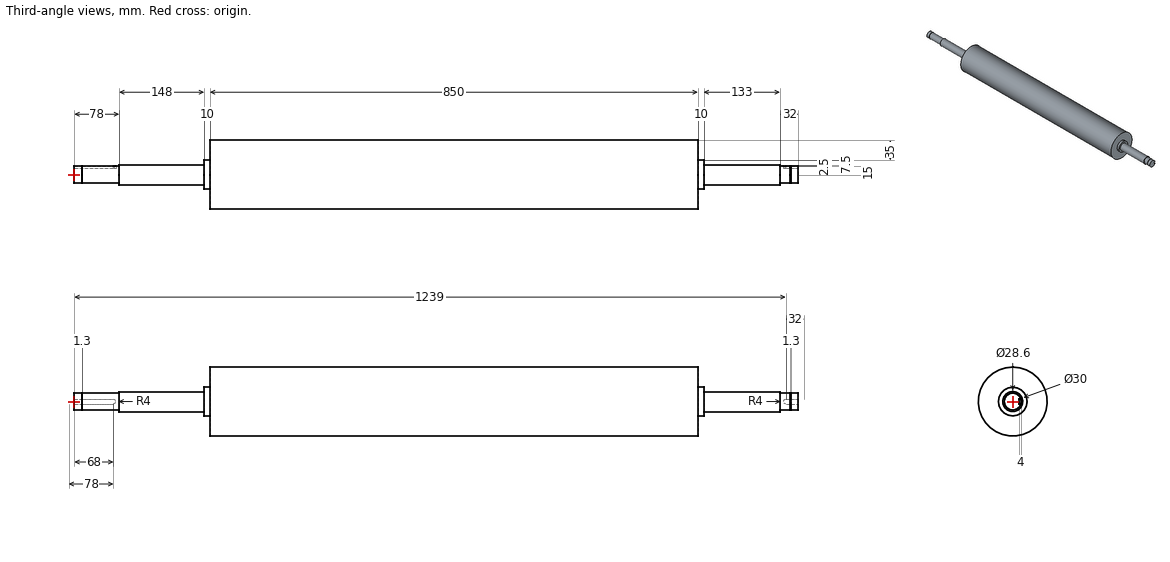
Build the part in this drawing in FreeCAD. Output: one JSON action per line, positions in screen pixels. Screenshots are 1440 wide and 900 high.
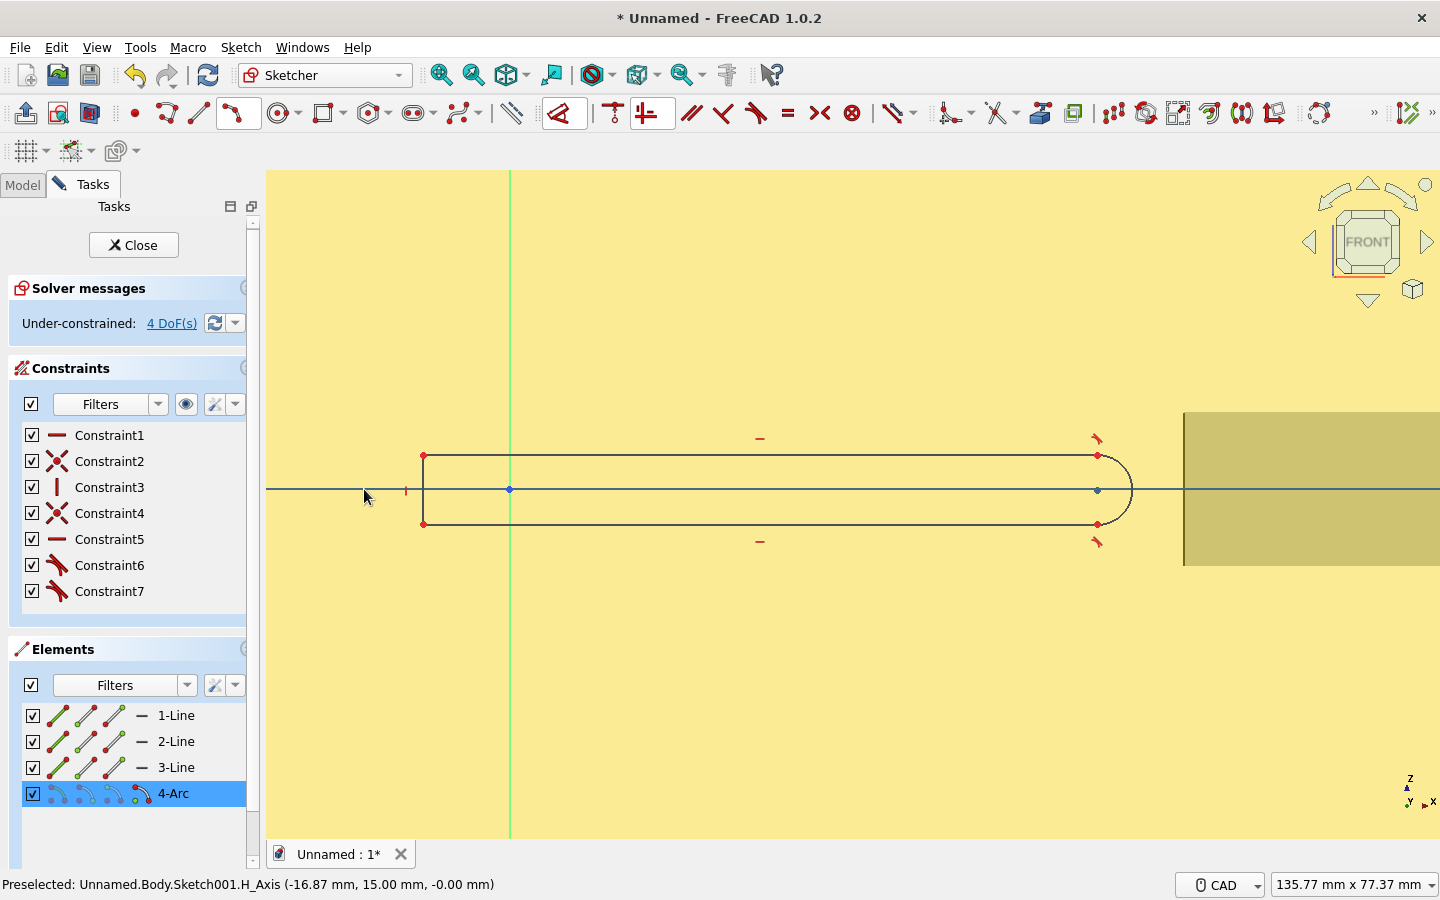
{"action": "left_click", "coordinate": [614, 114]}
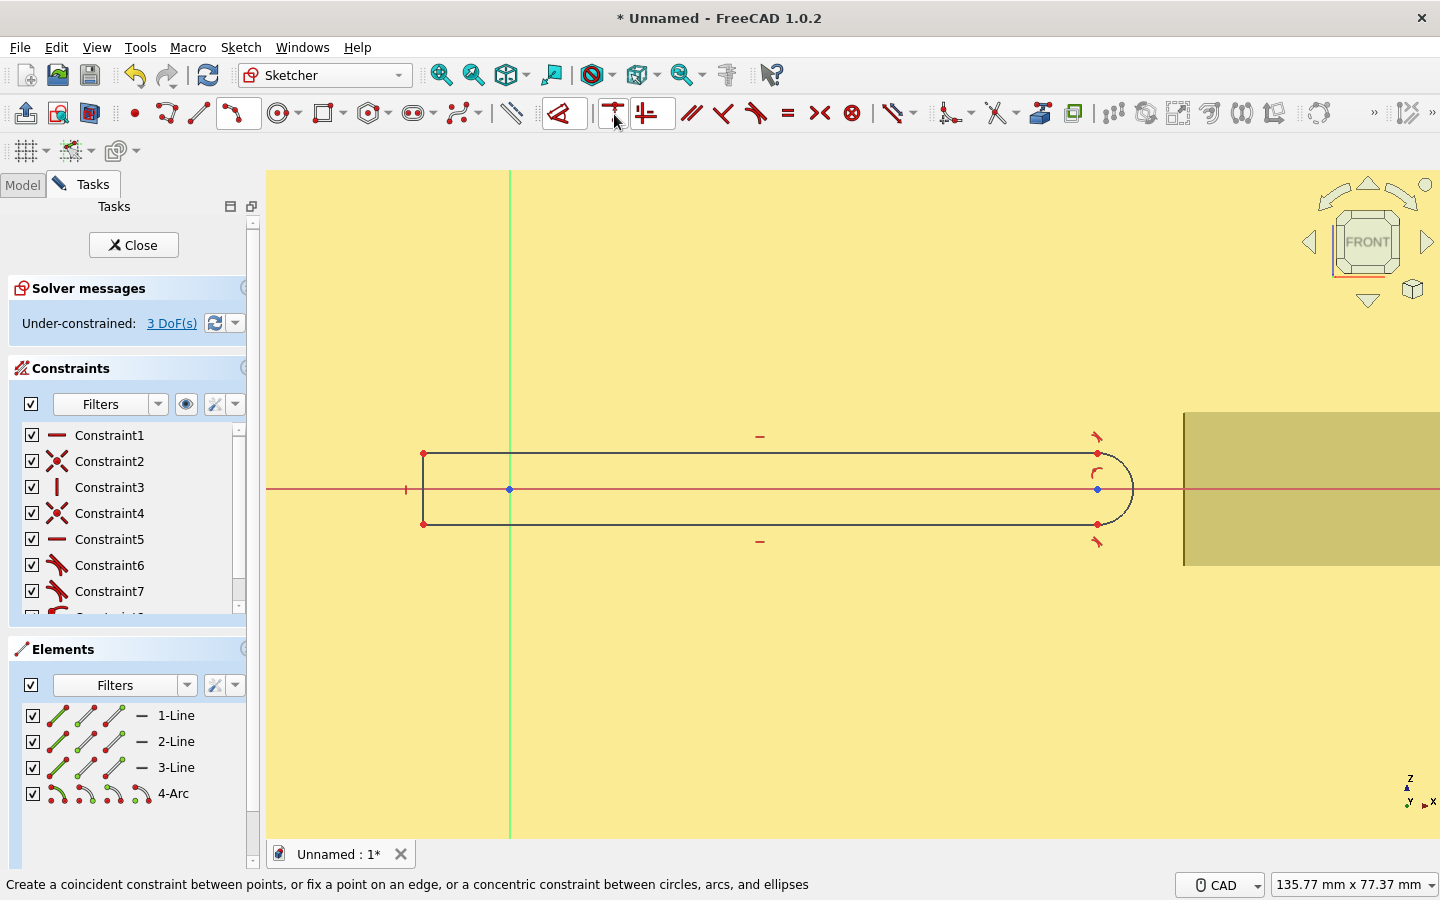
{"action": "left_click", "coordinate": [1126, 510]}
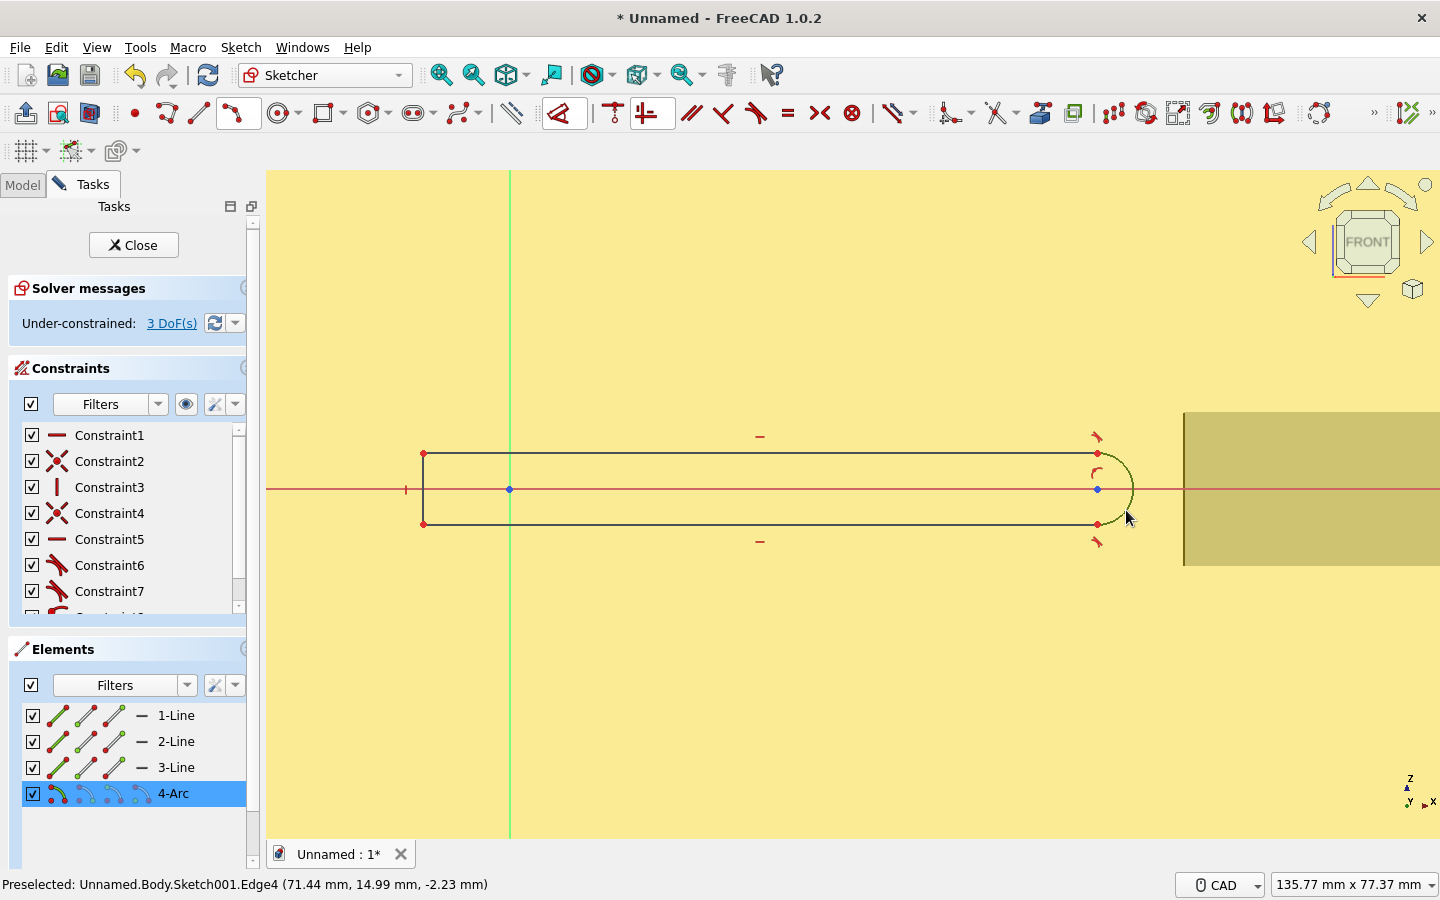
{"action": "key", "text": "k r"}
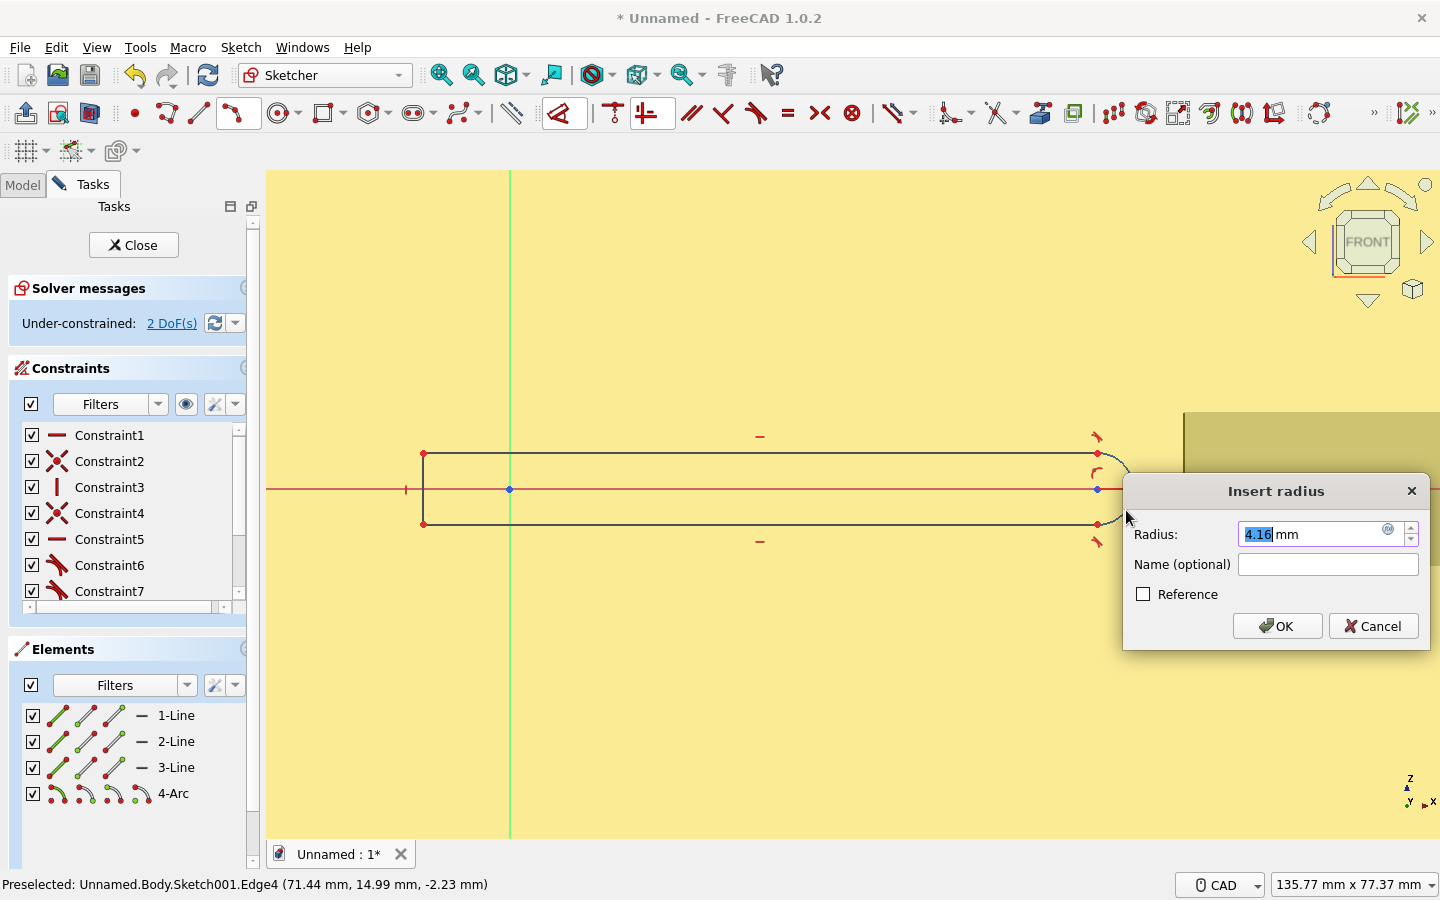
{"action": "type", "text": "4"}
{"action": "key", "text": "Return"}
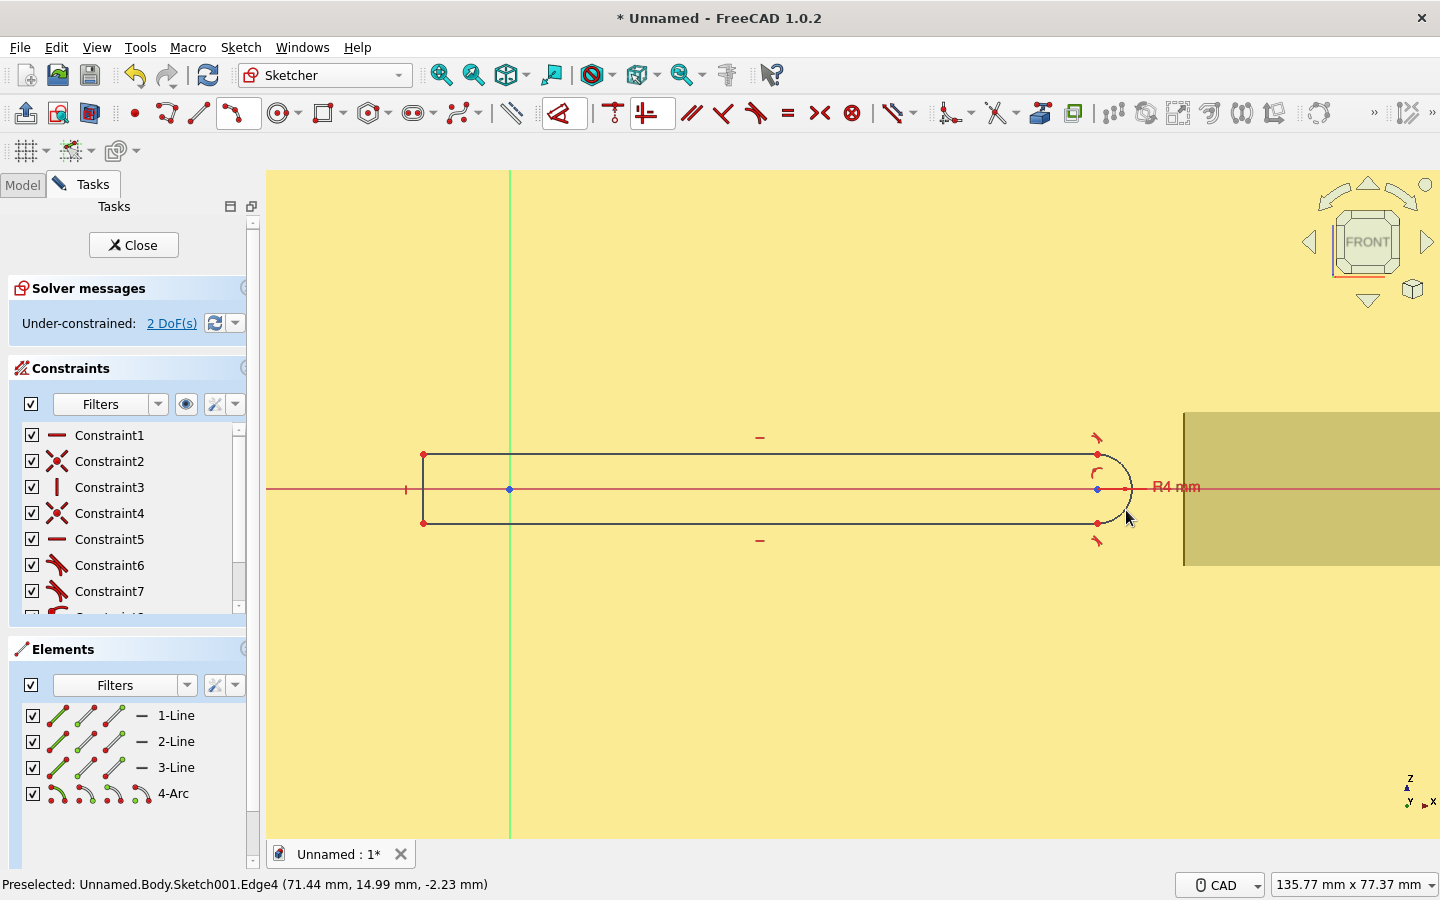
{"action": "left_click", "coordinate": [895, 524]}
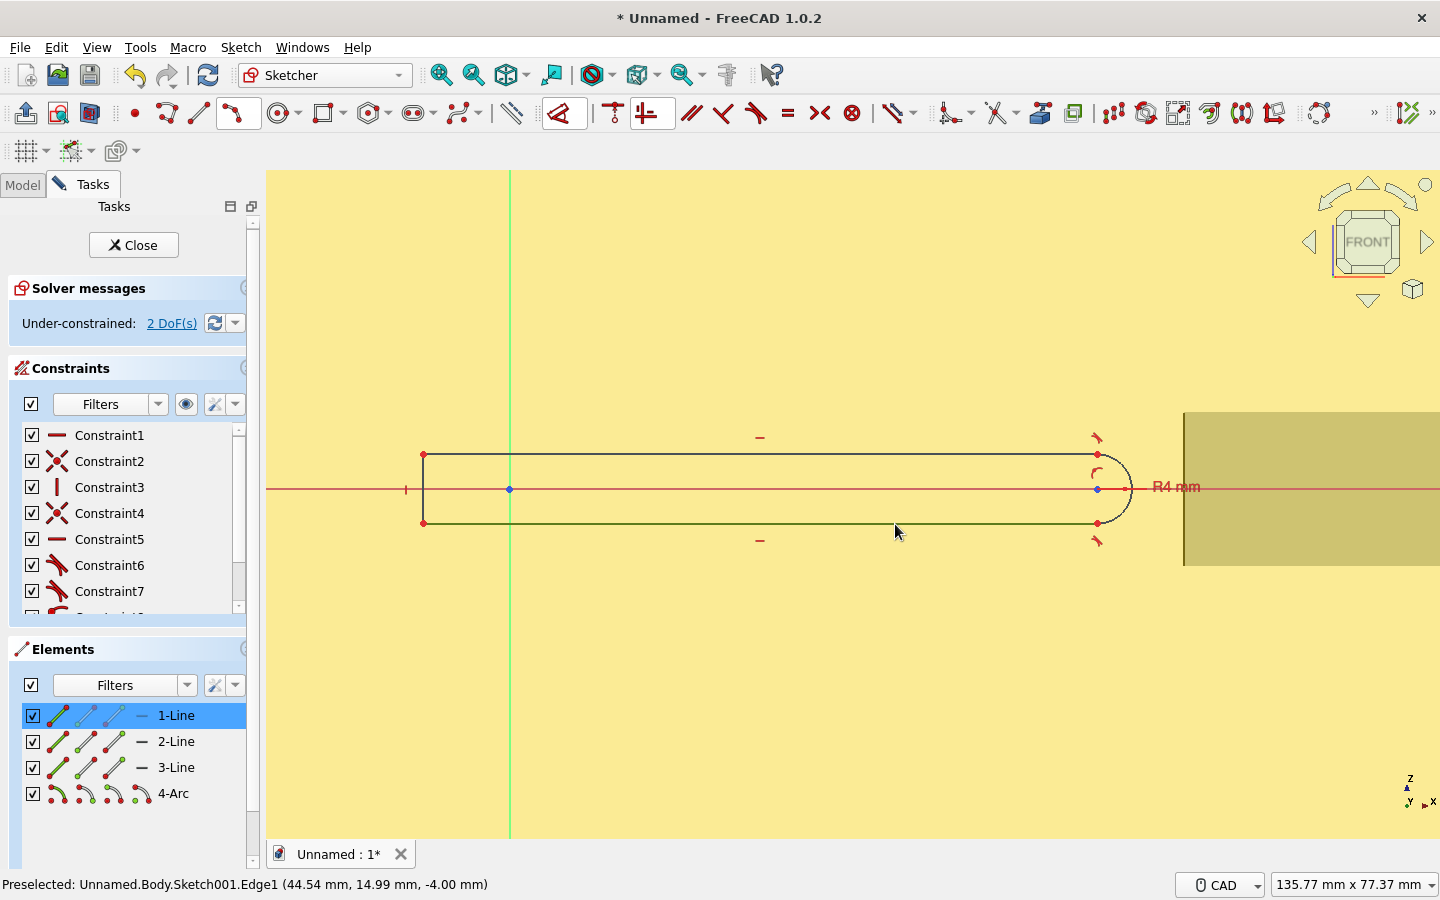
{"action": "left_click", "coordinate": [582, 114]}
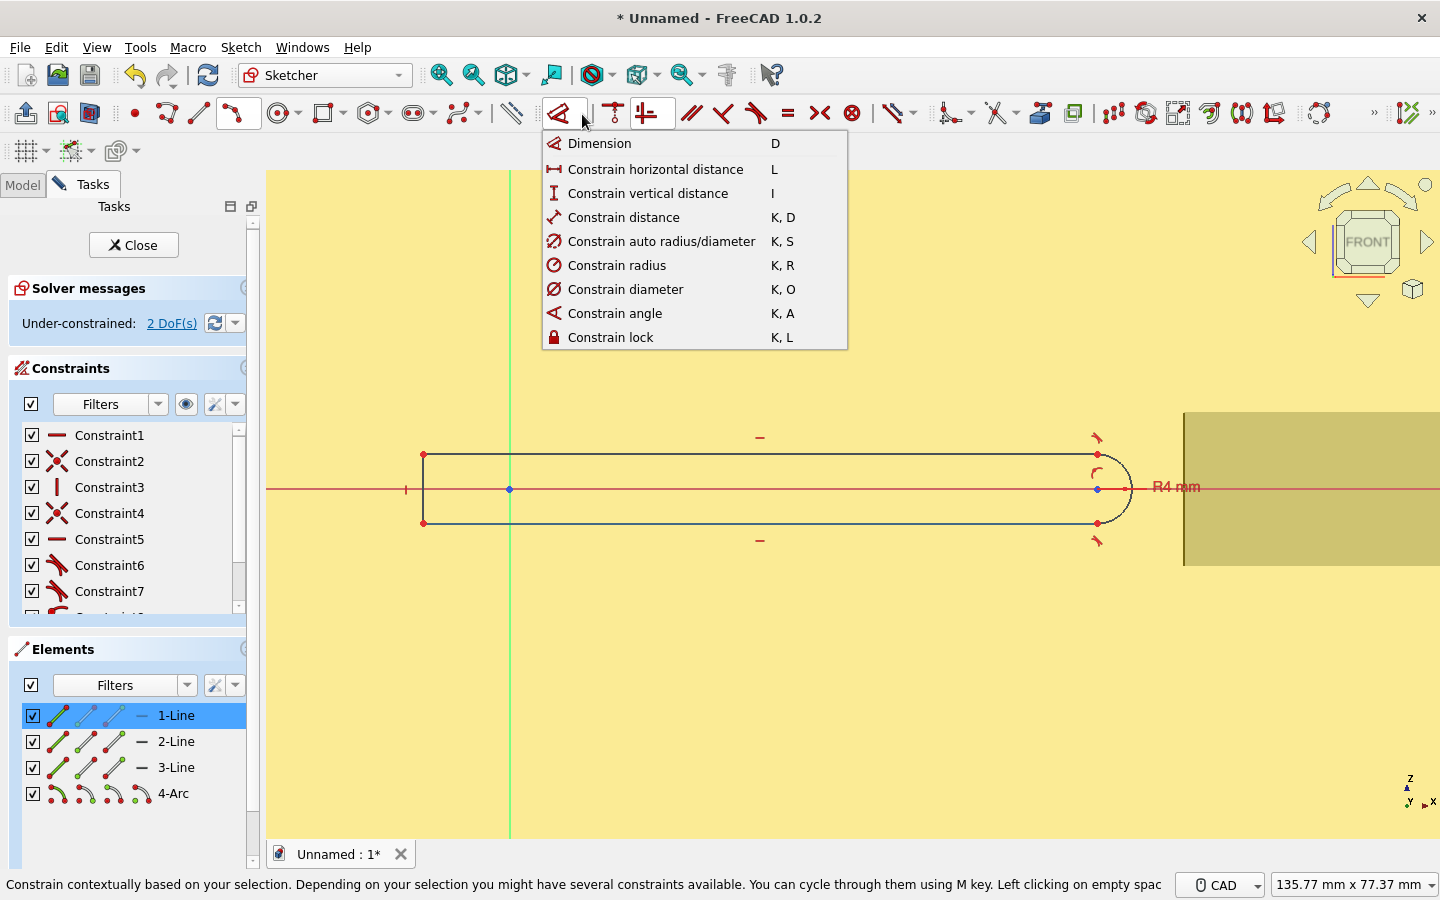
{"action": "left_click", "coordinate": [695, 169]}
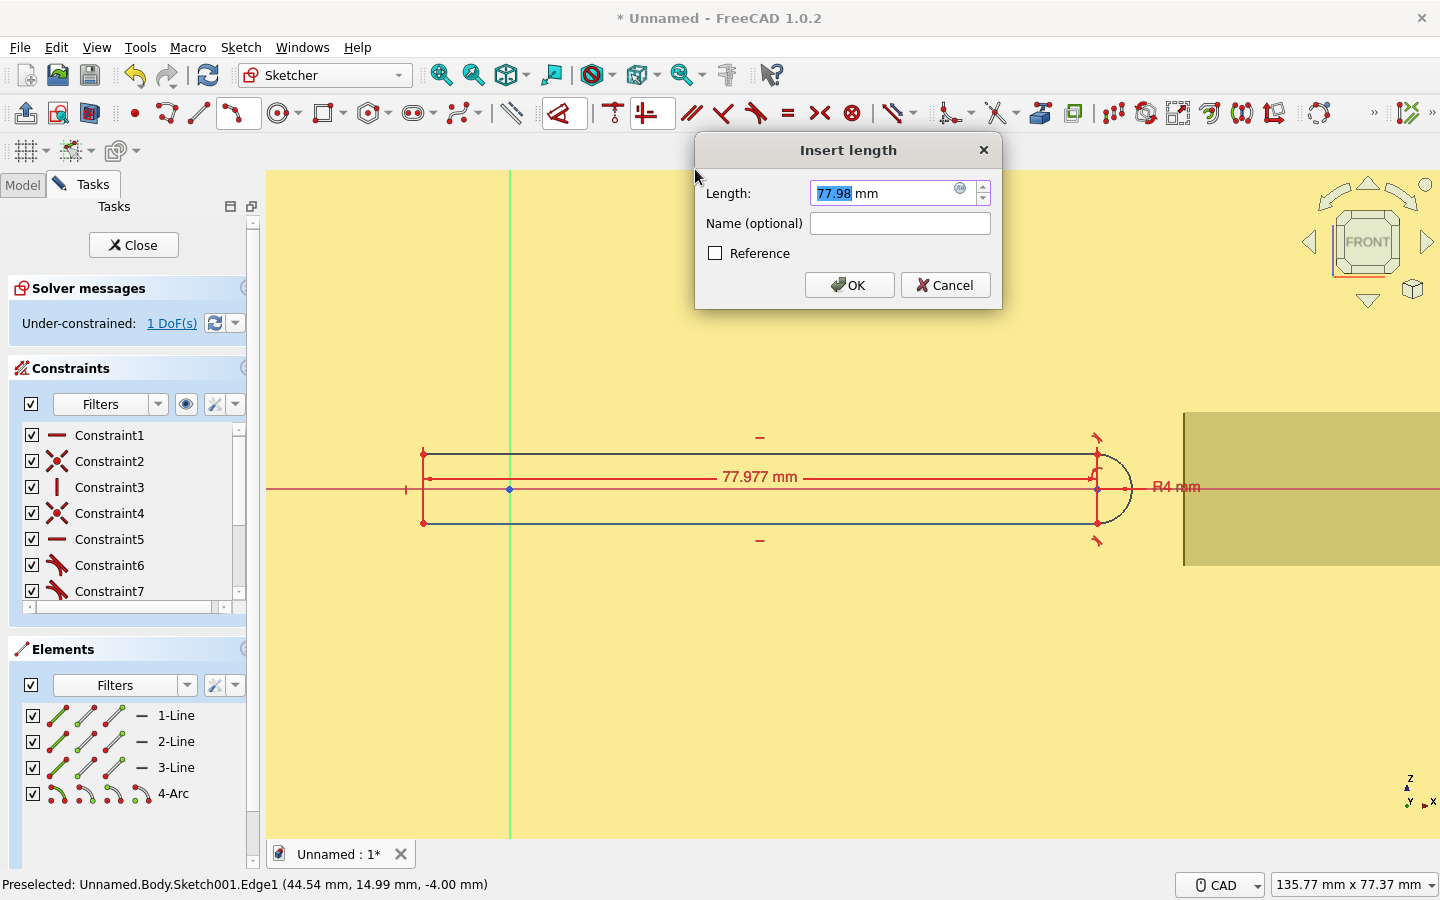
{"action": "type", "text": "78"}
{"action": "key", "text": "Return"}